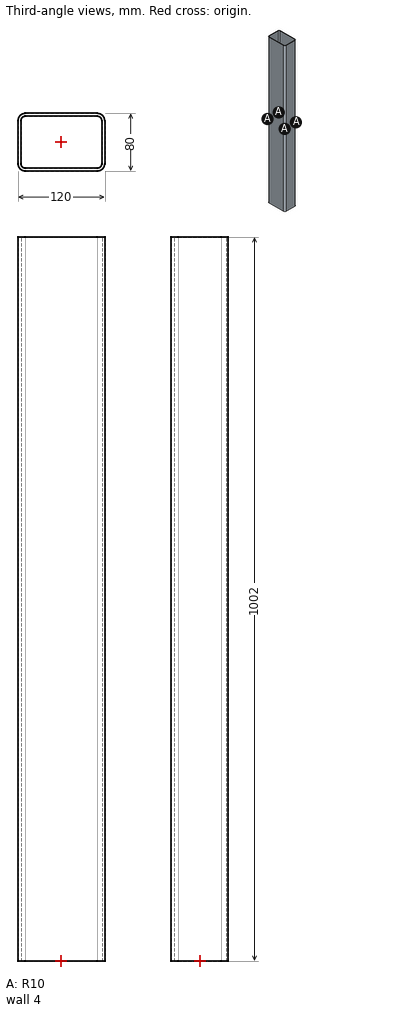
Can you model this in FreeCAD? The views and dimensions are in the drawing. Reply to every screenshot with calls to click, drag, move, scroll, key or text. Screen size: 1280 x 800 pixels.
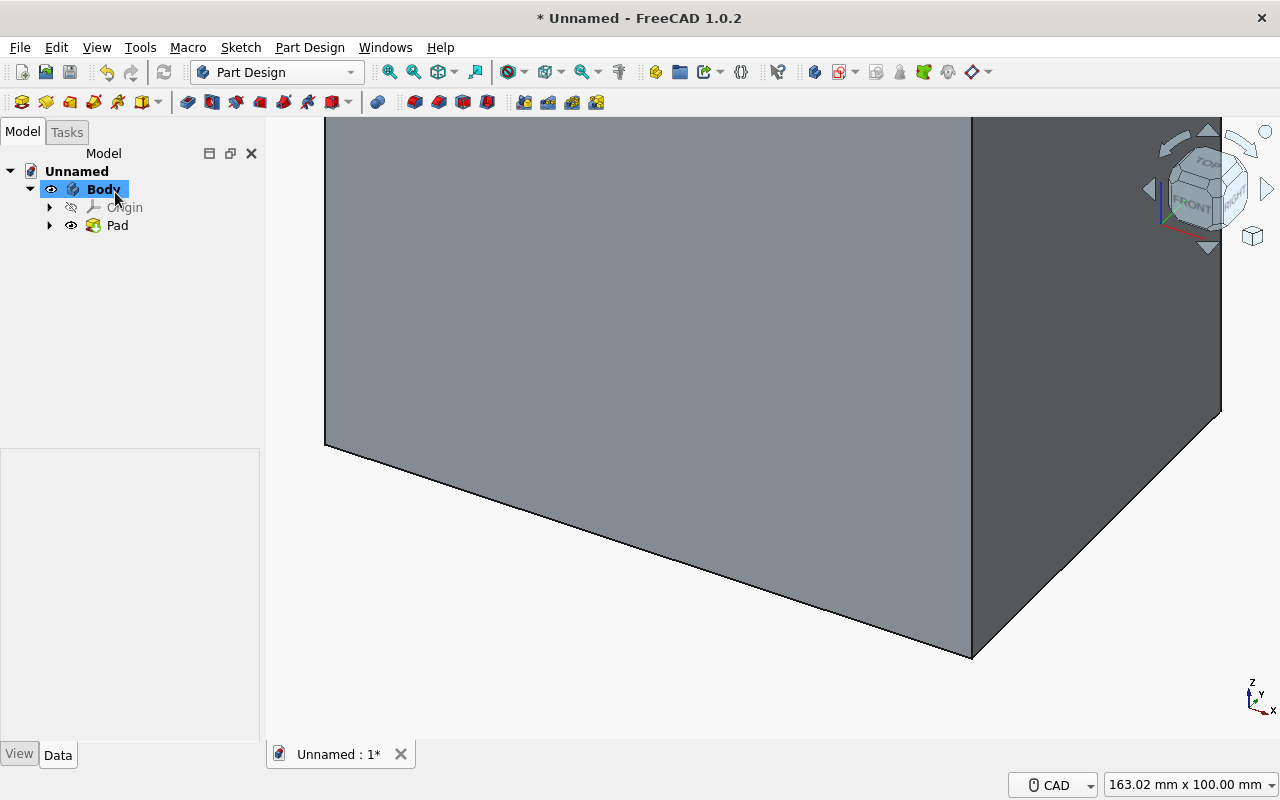
click(390, 72)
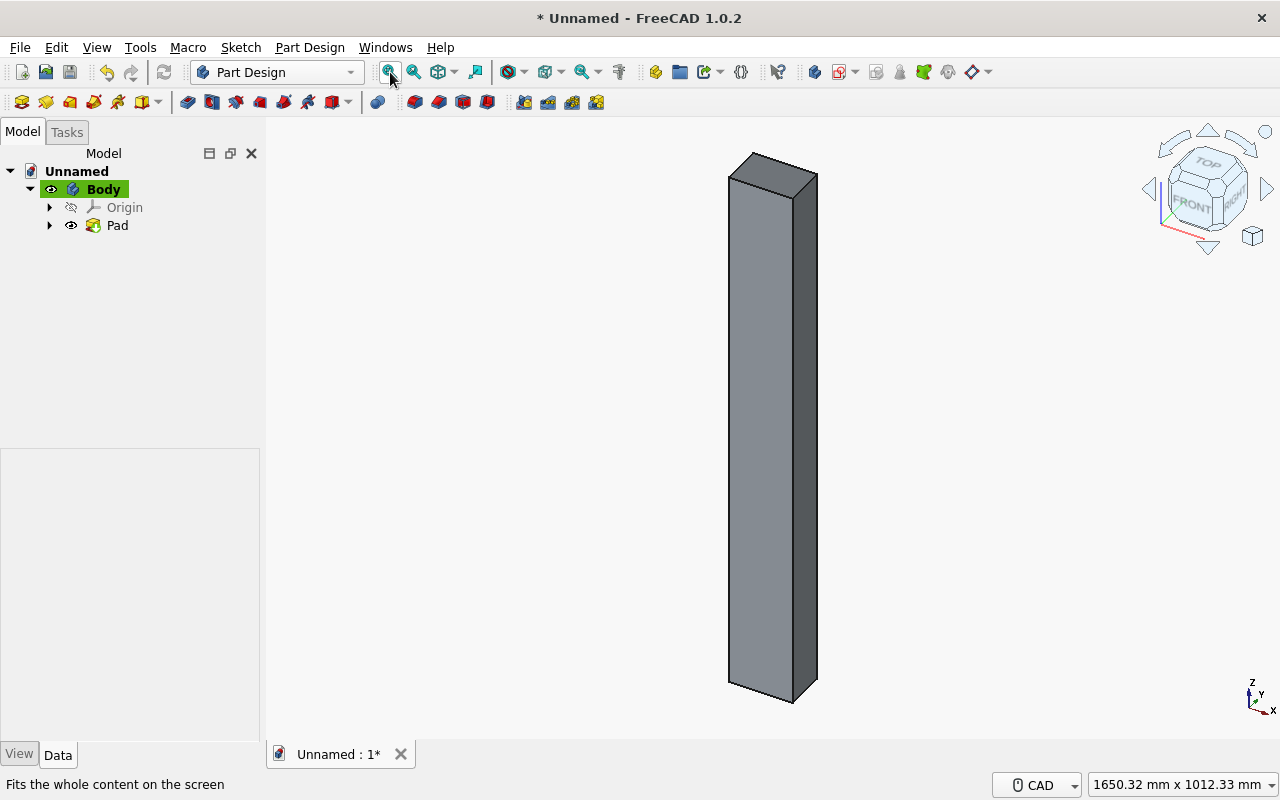
click(793, 450)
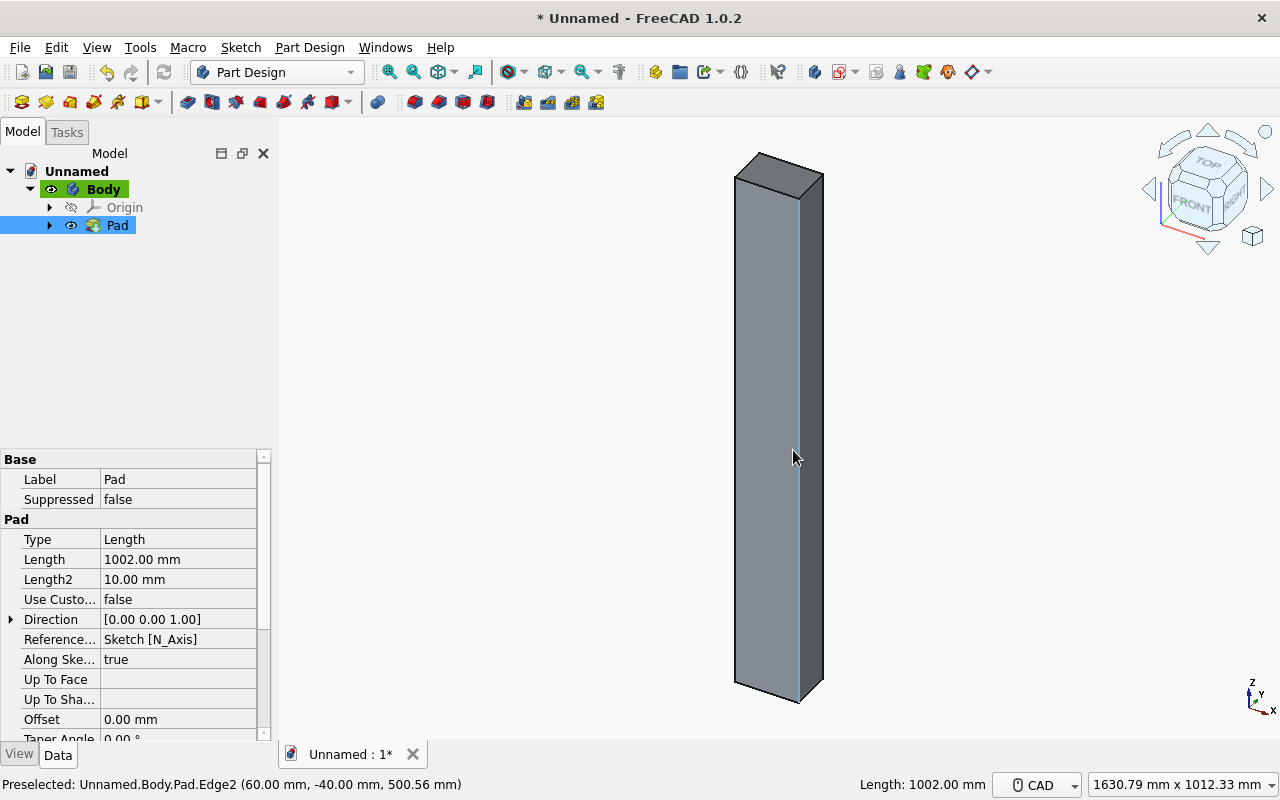
key(0)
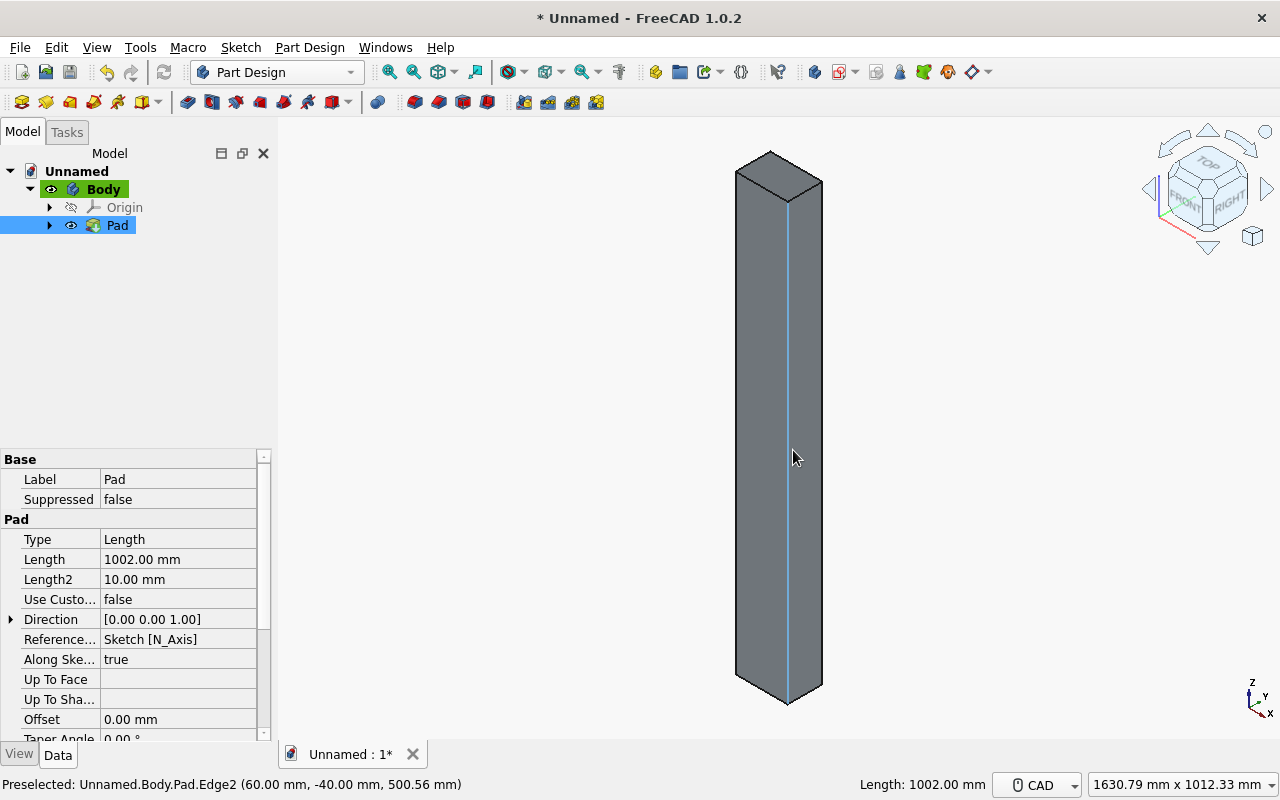
key(2)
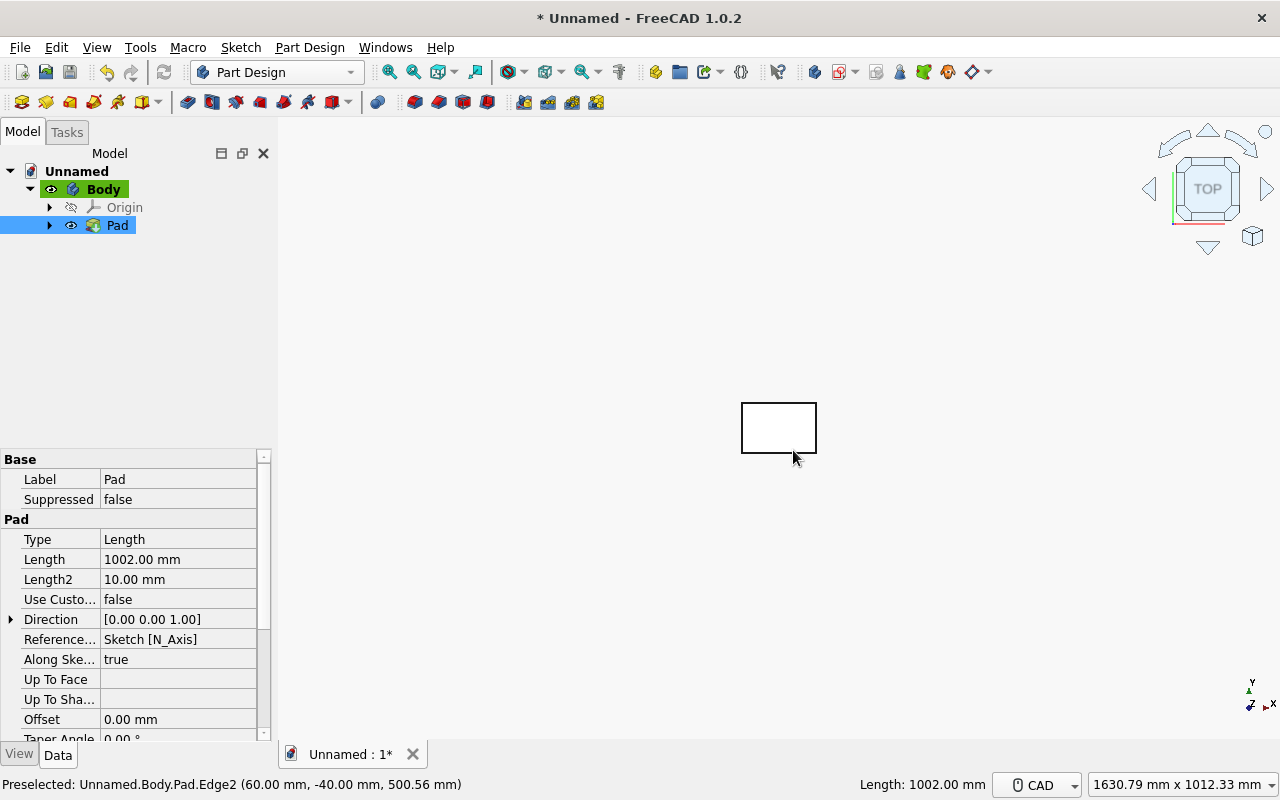
click(390, 72)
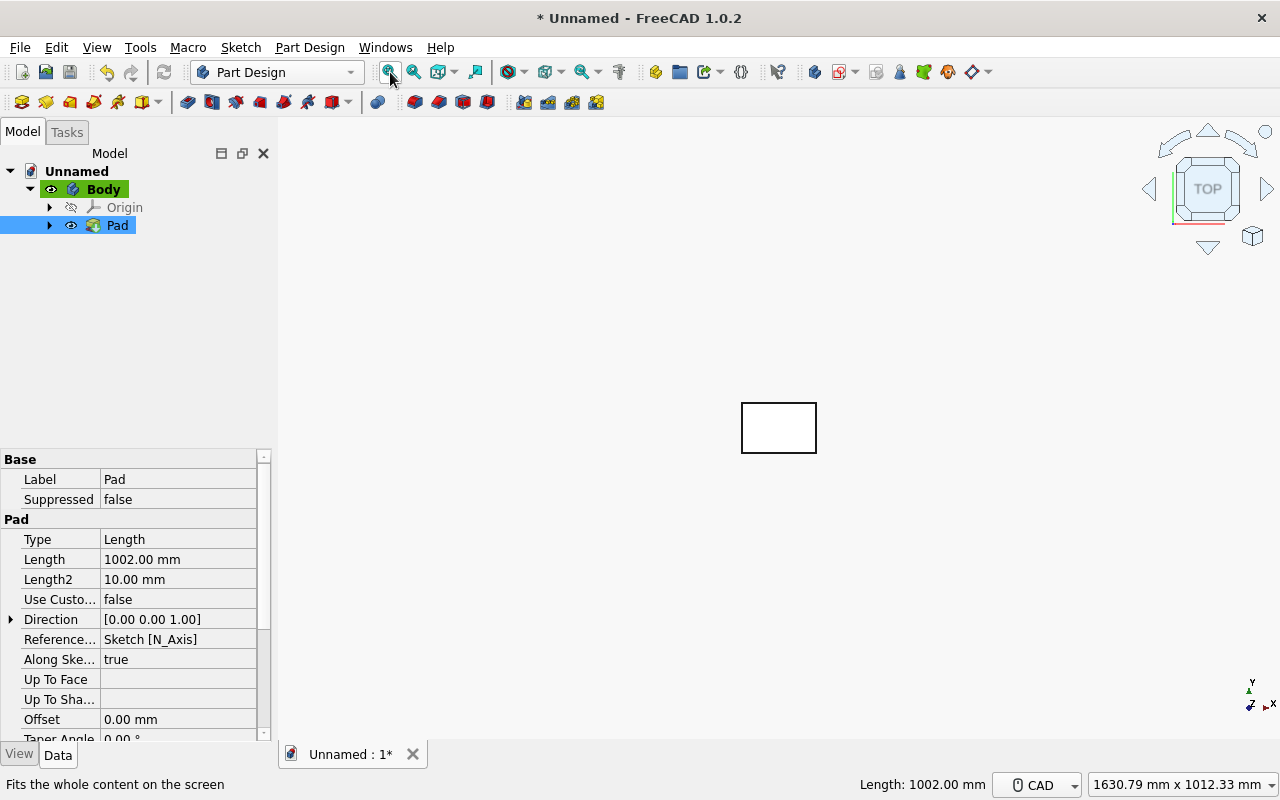
key(1)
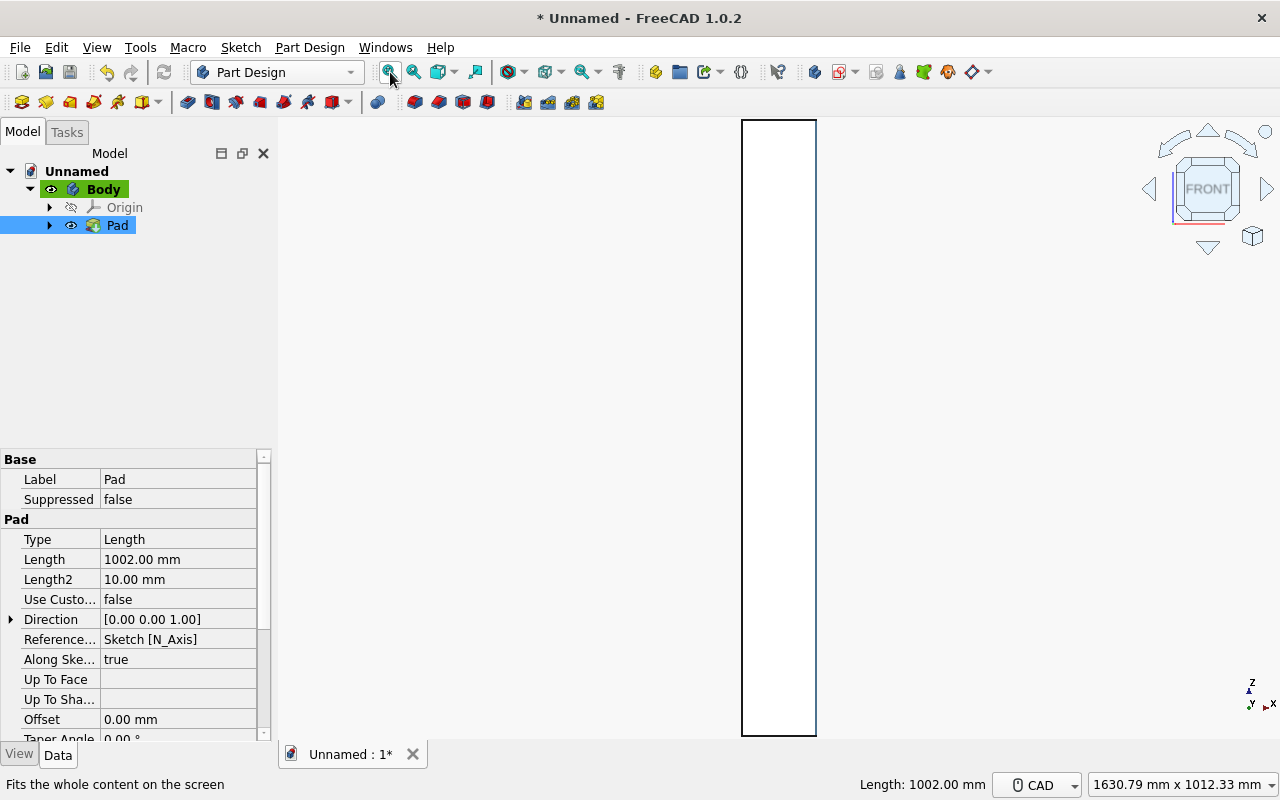
click(742, 427, ctrl)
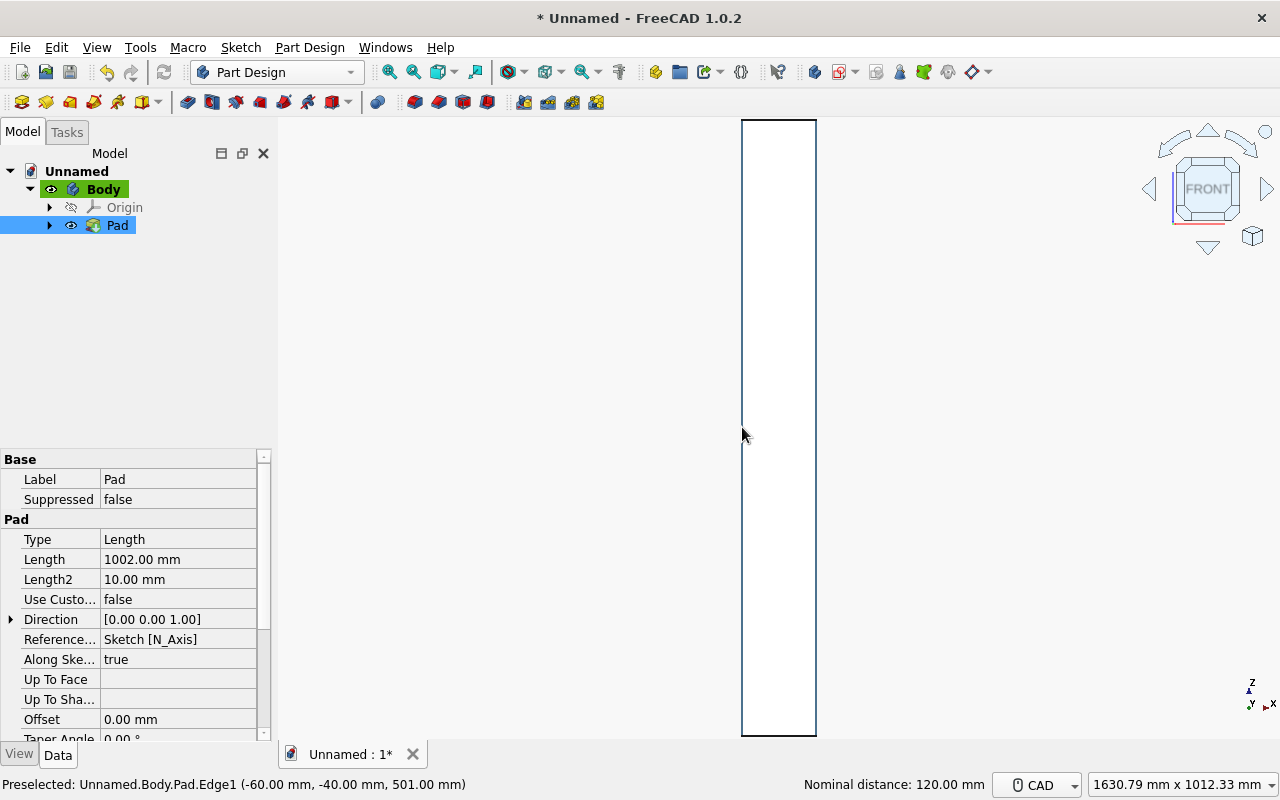
key(3)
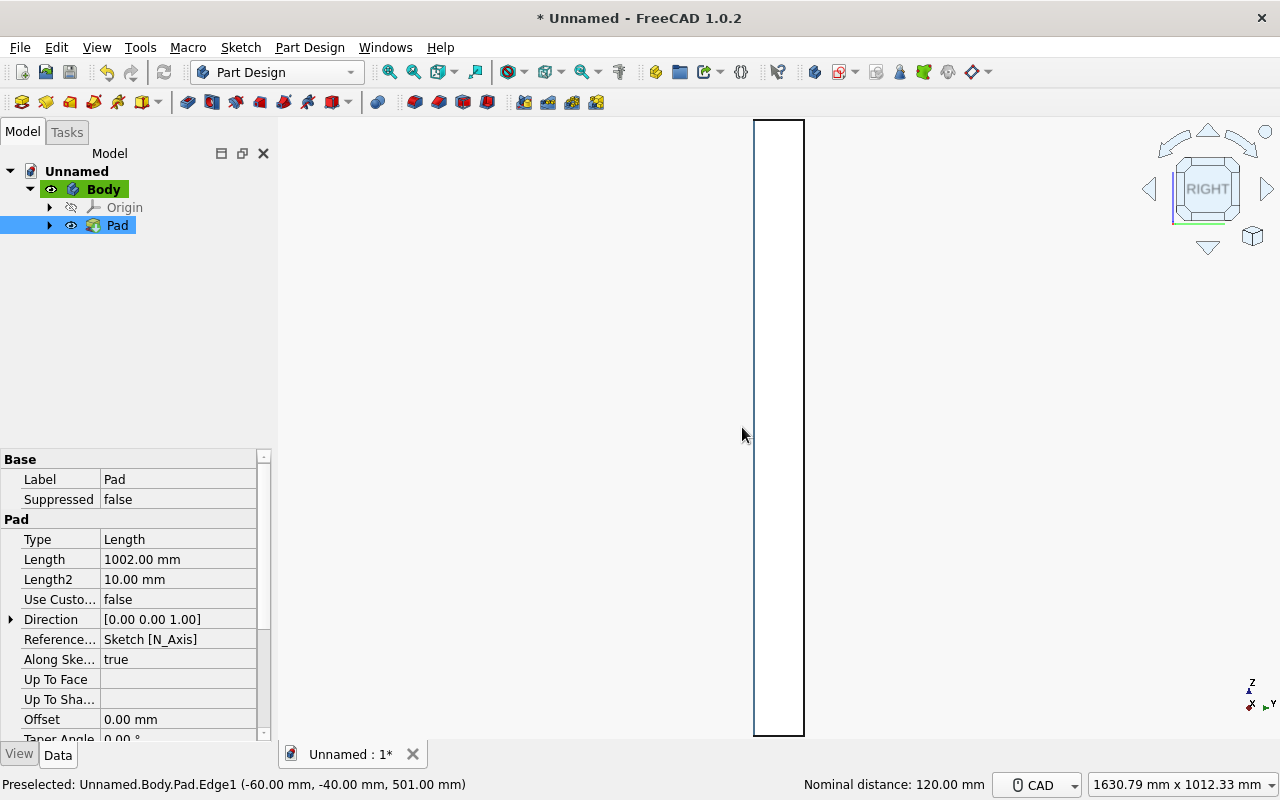
click(804, 427, ctrl)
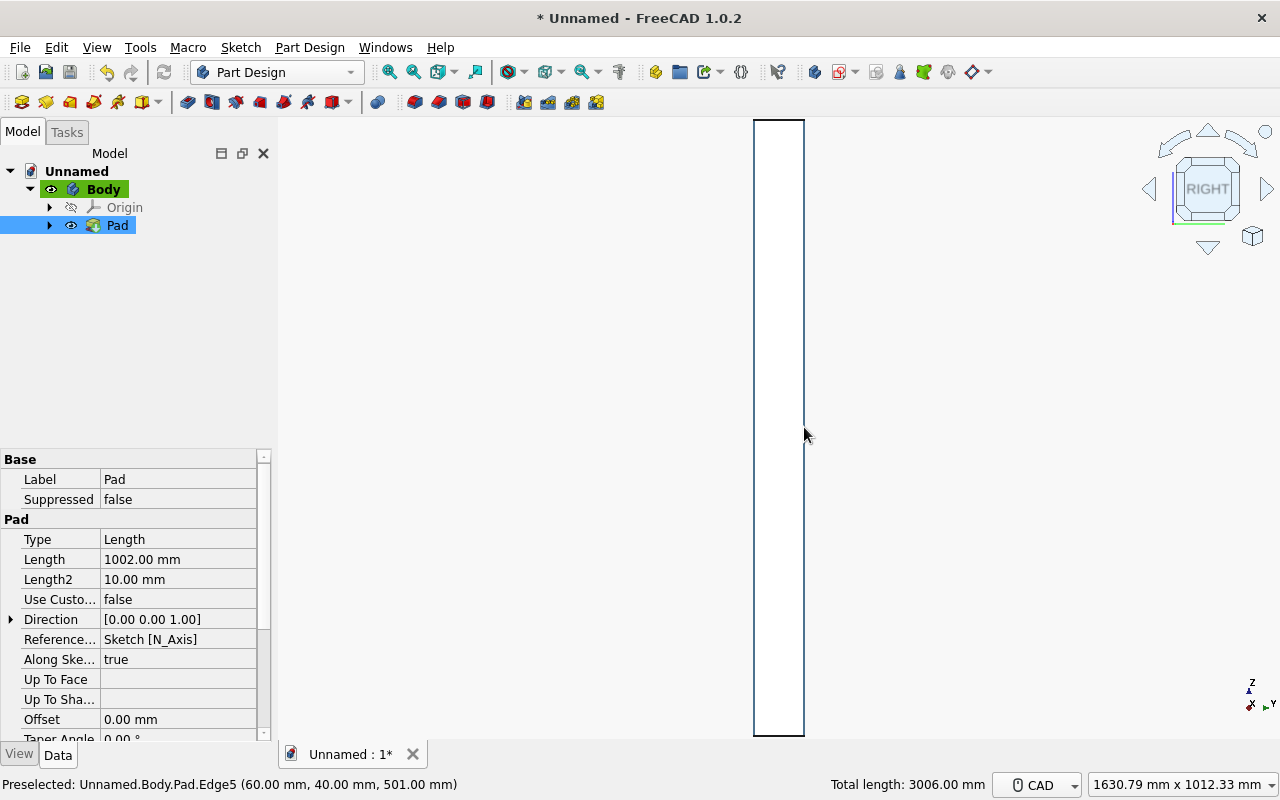
key(5)